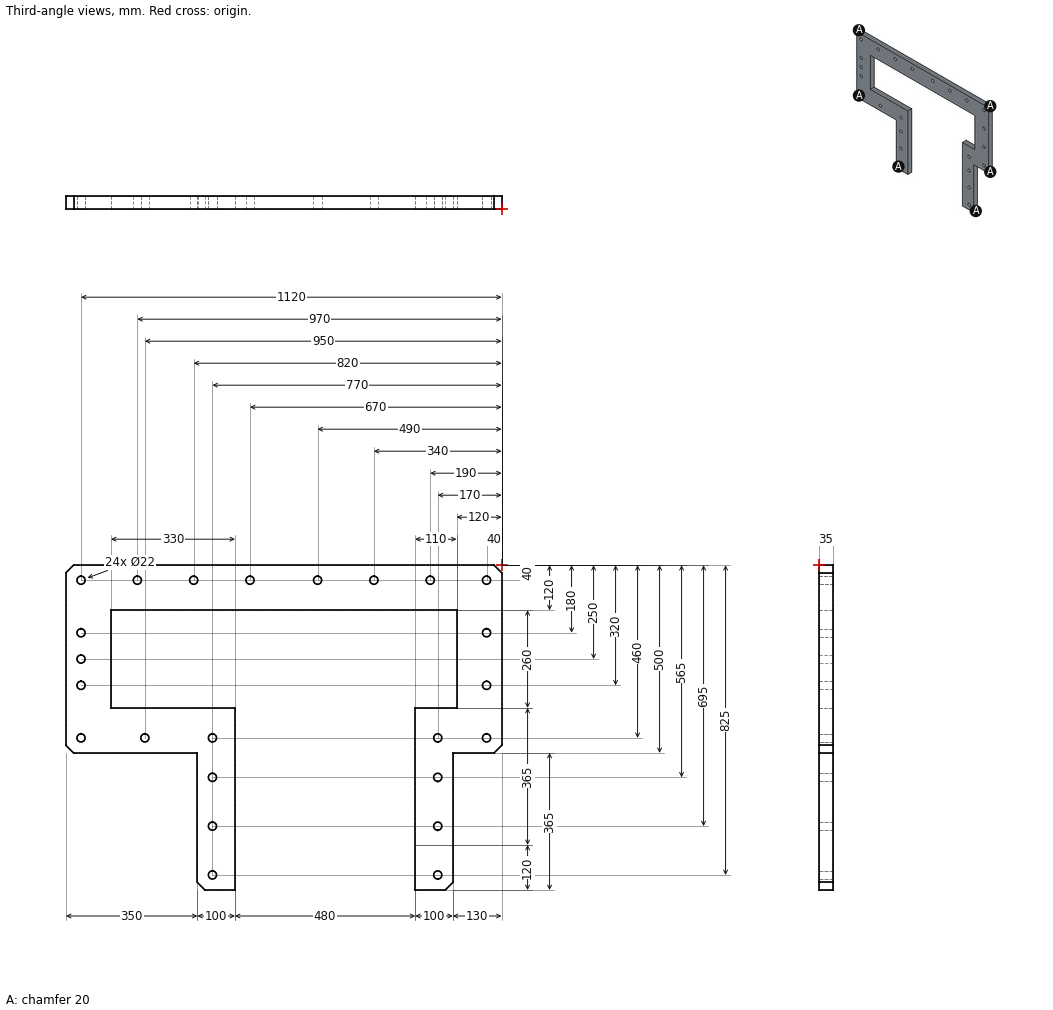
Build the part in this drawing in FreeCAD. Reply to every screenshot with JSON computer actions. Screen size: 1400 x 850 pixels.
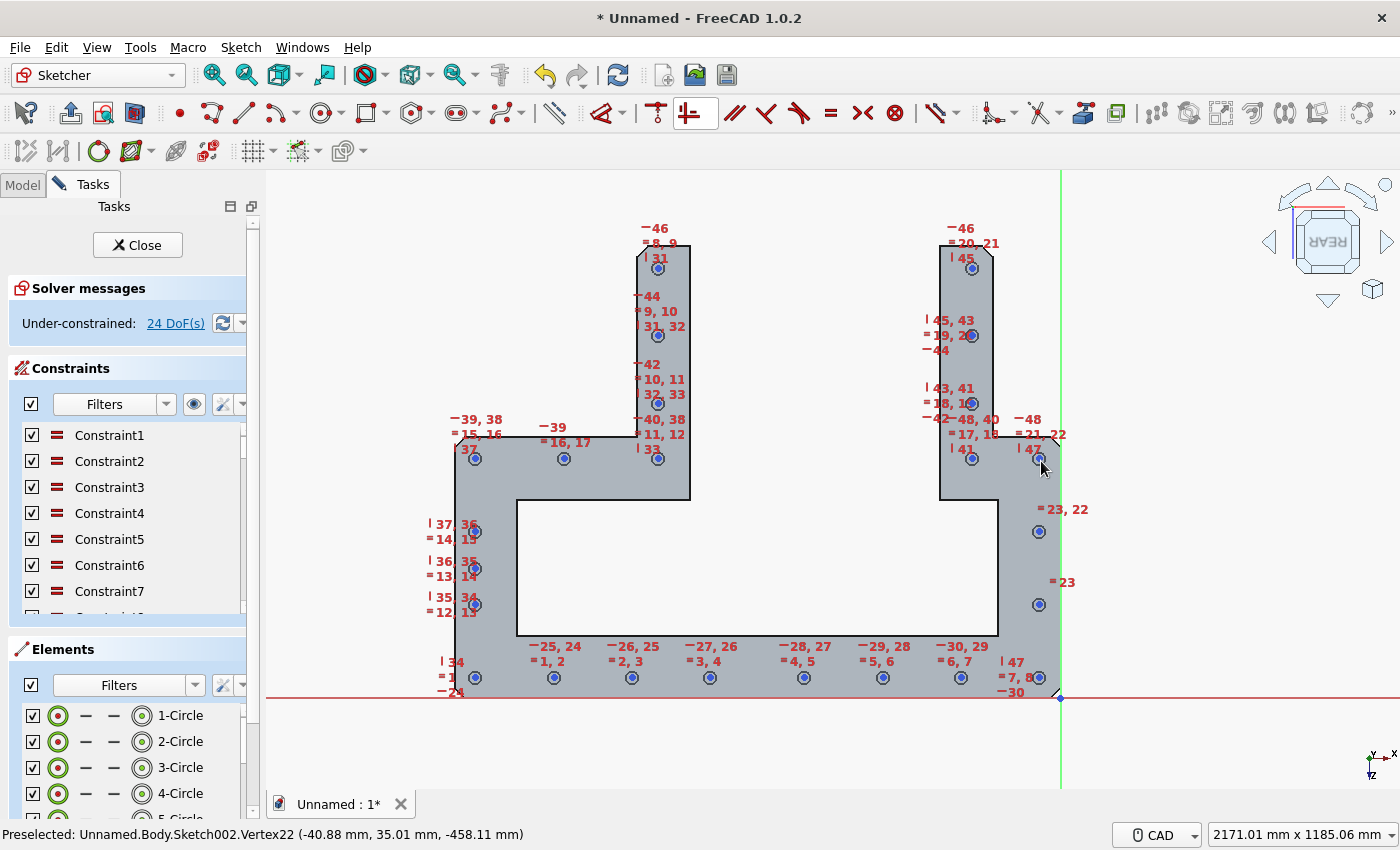
{"action": "left_click", "coordinate": [1039, 459]}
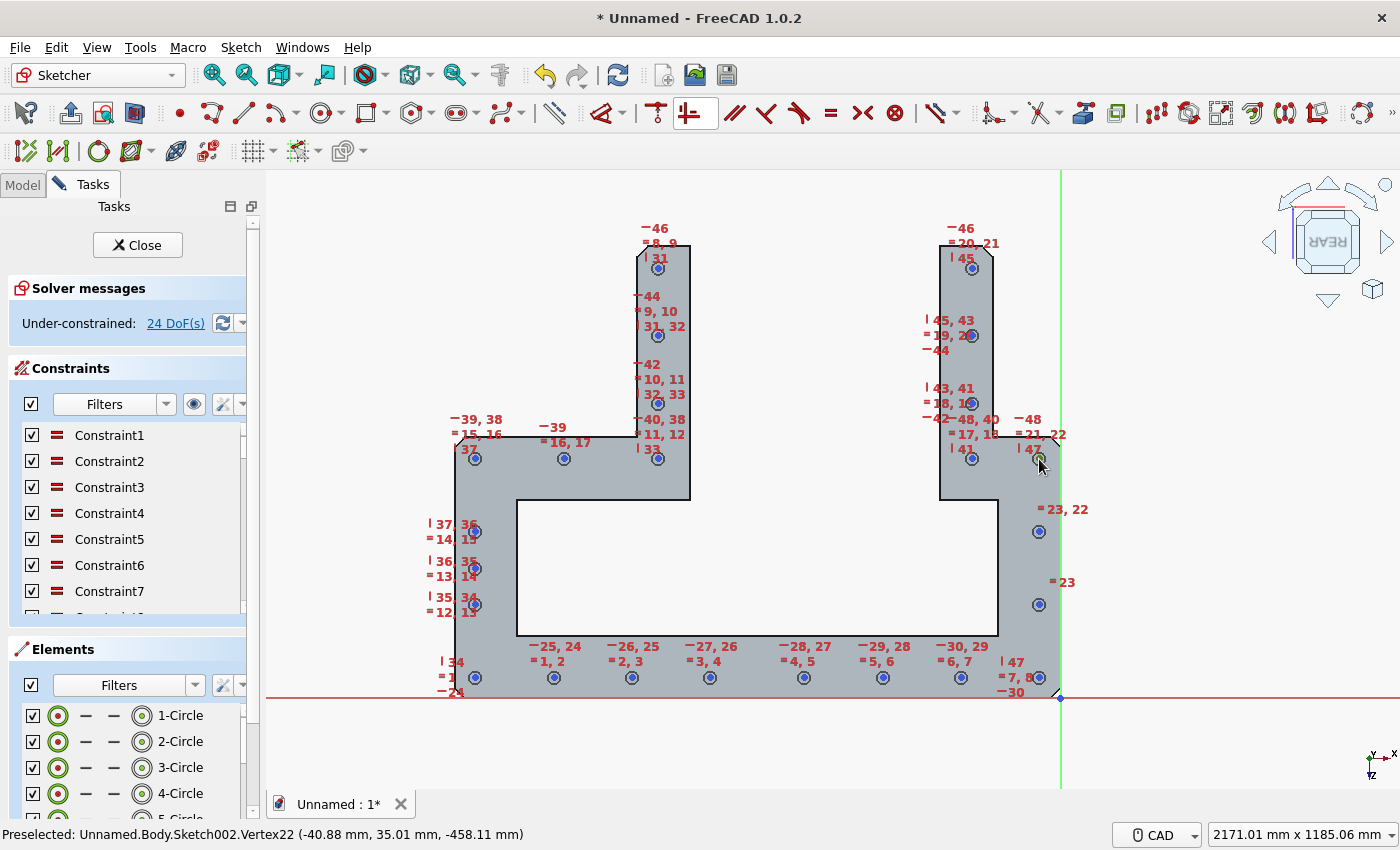
{"action": "left_click", "coordinate": [1039, 532]}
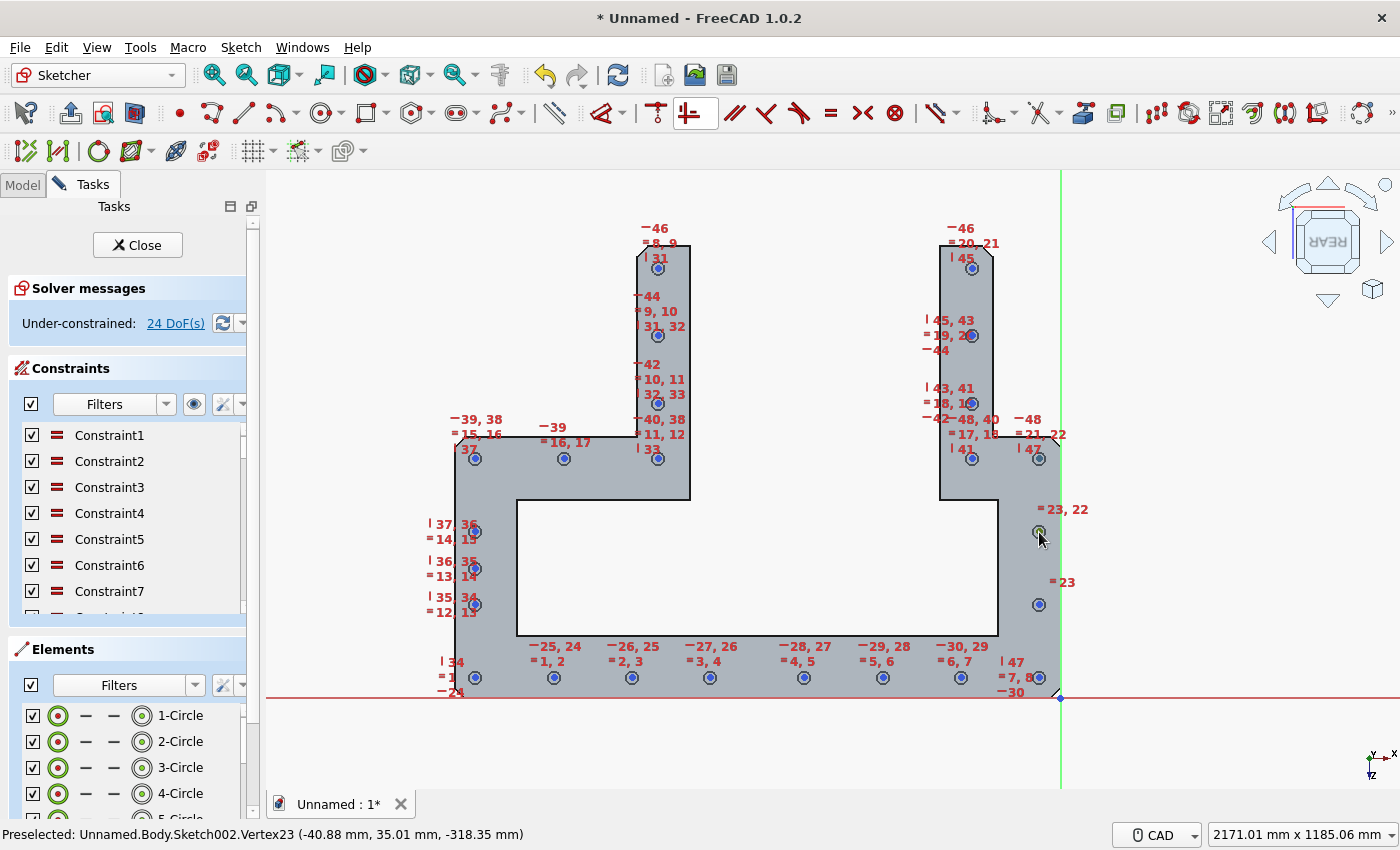
{"action": "key", "text": "v"}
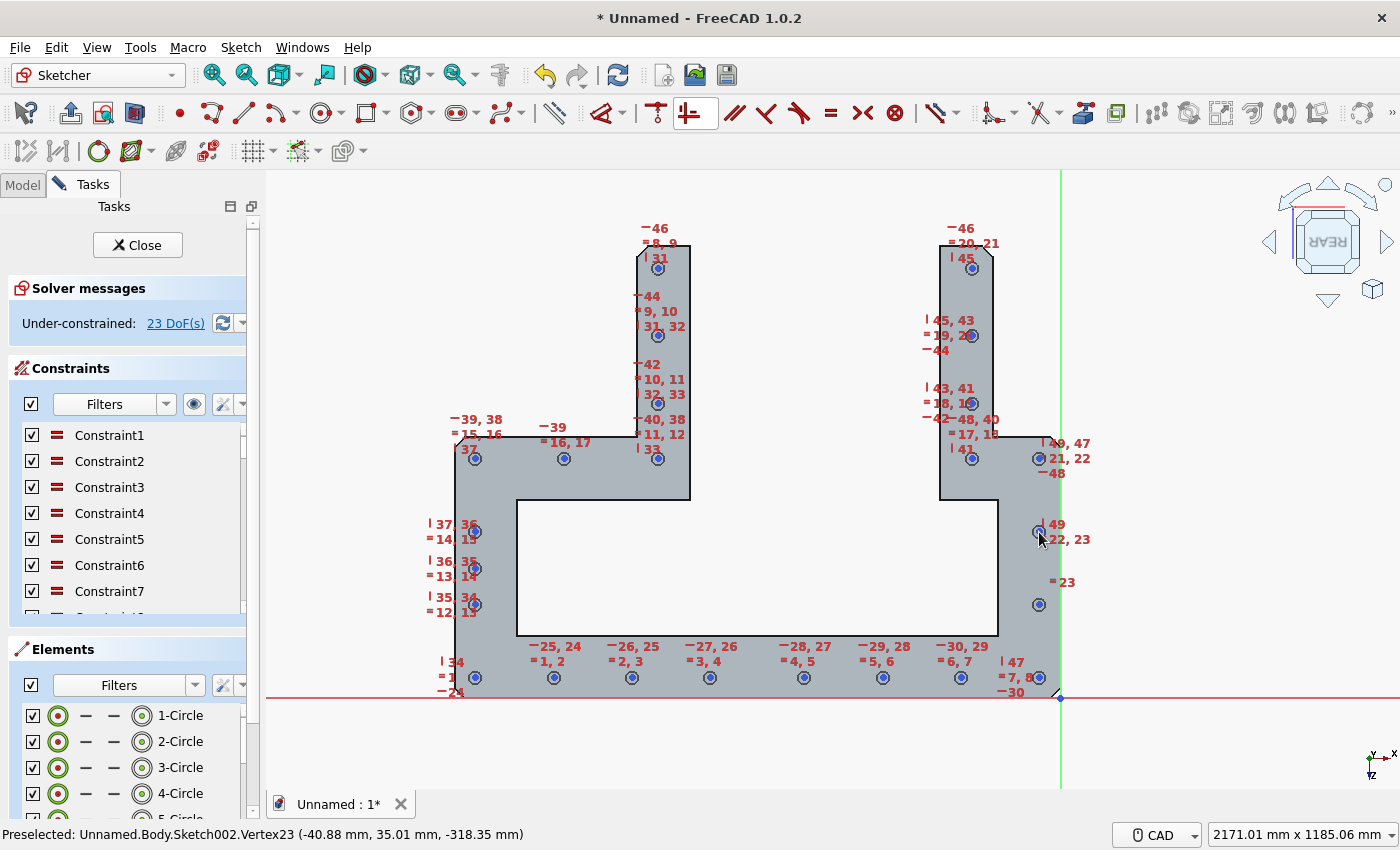
{"action": "left_click", "coordinate": [1039, 678]}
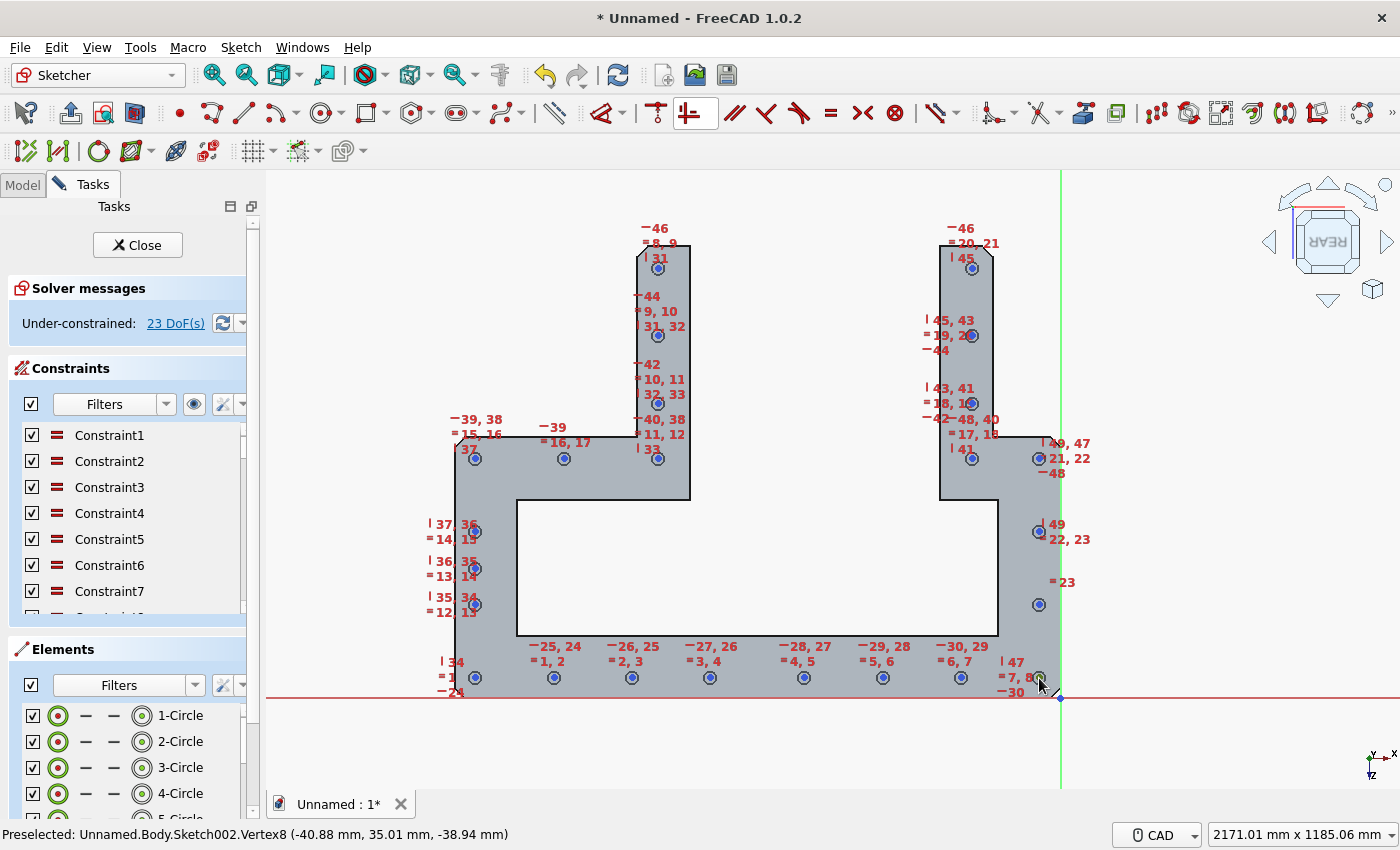
{"action": "left_click", "coordinate": [1039, 605]}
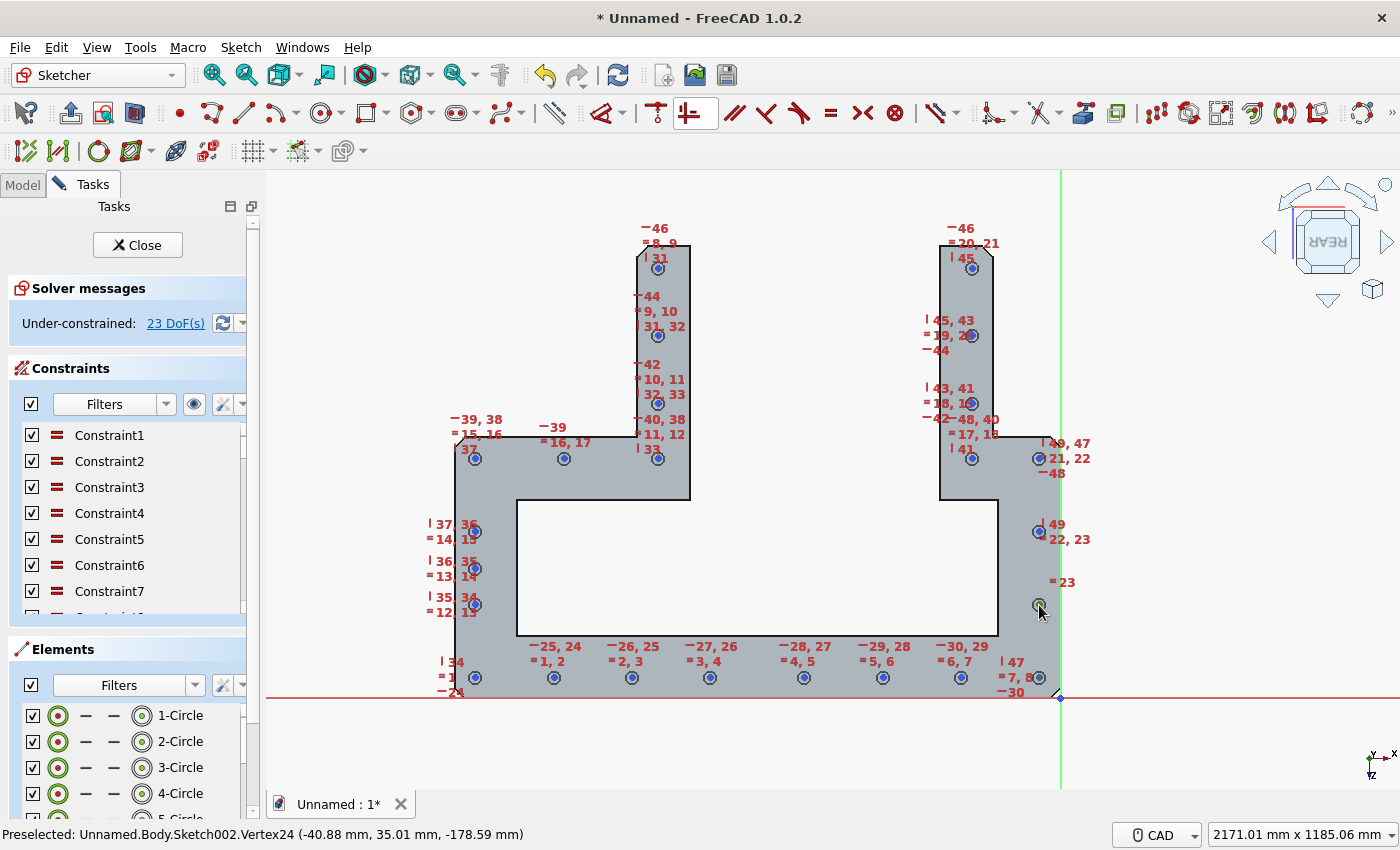
{"action": "key", "text": "v"}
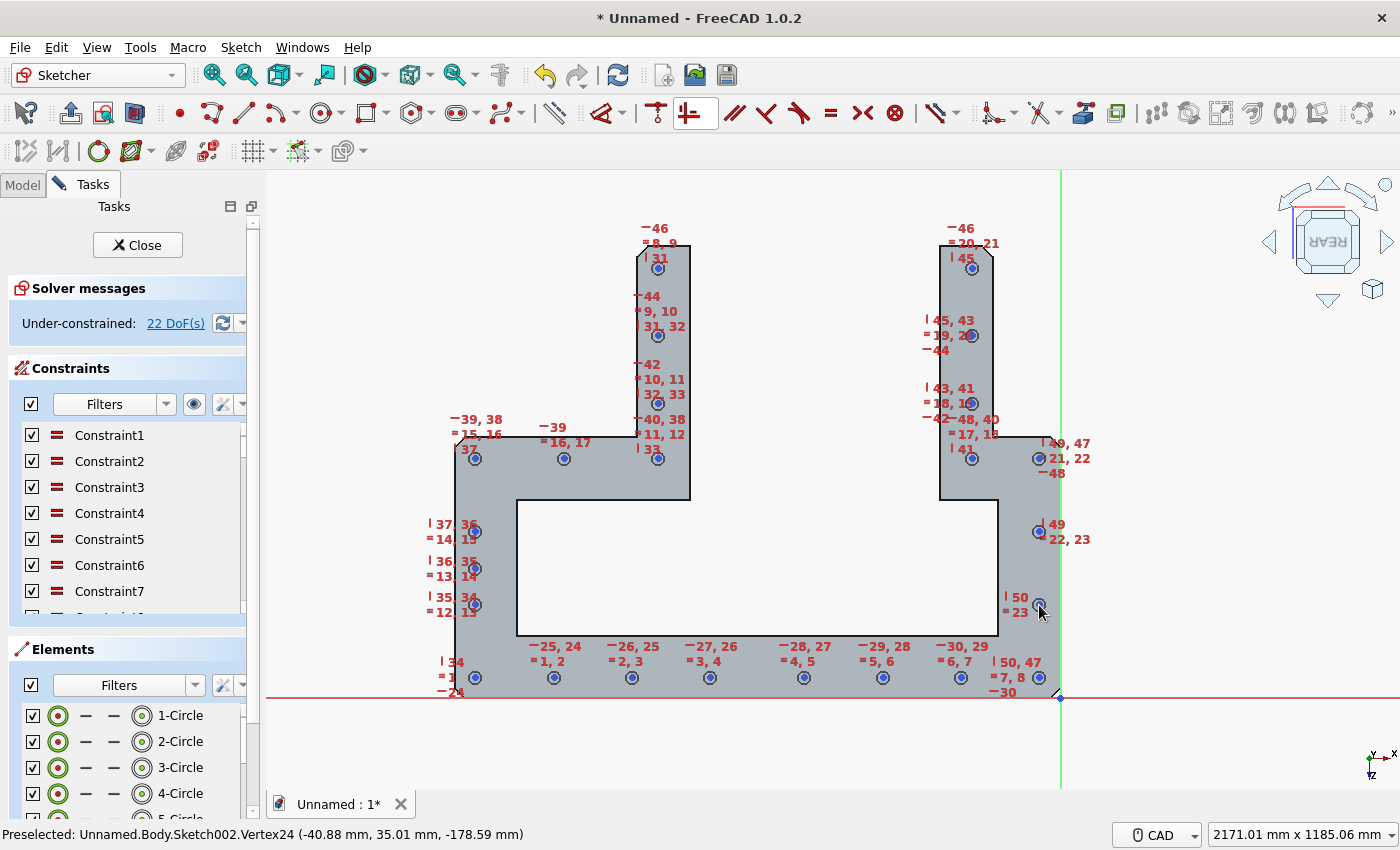
{"action": "left_click", "coordinate": [602, 114]}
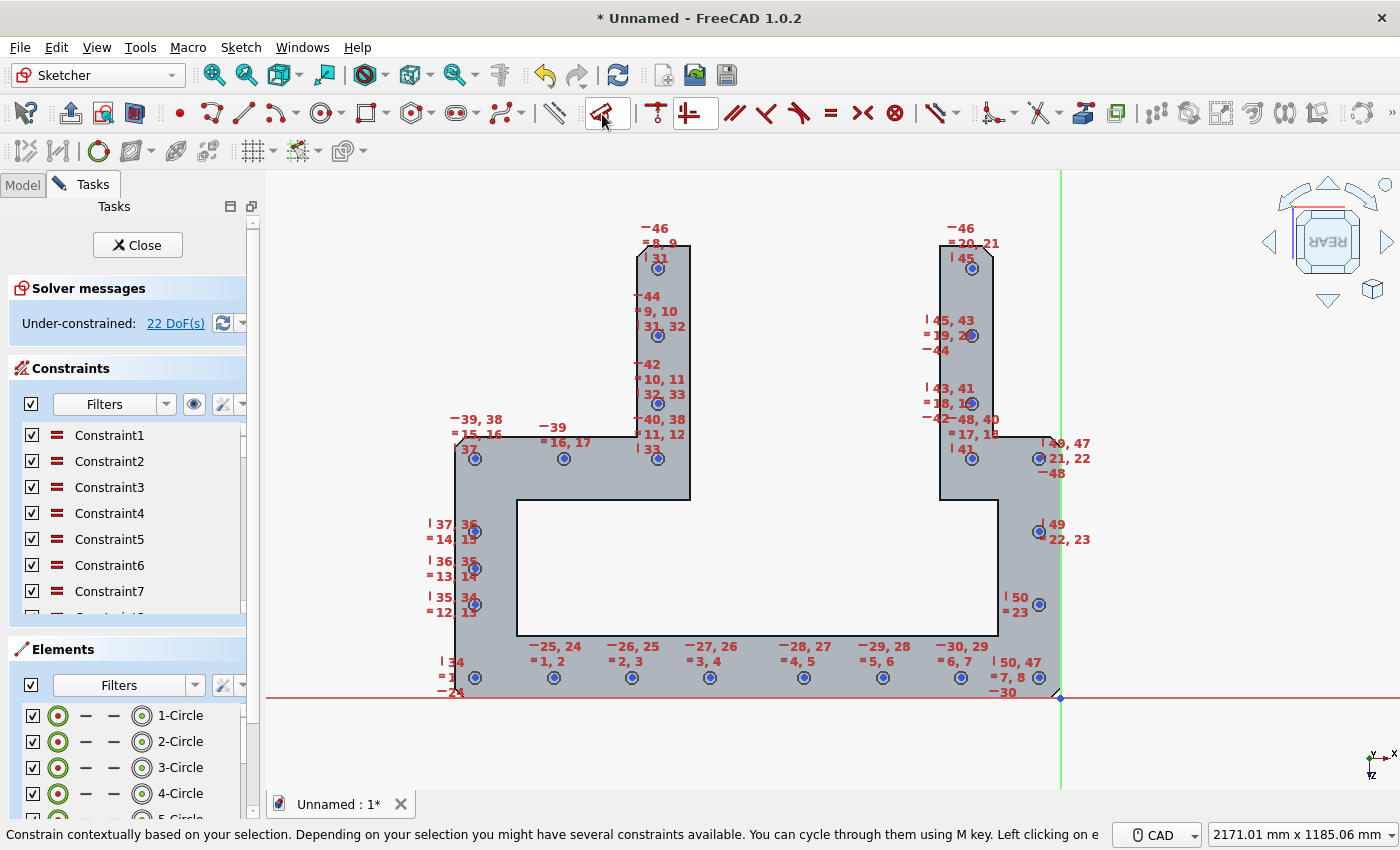
{"action": "scroll", "coordinate": [469, 678], "scroll_direction": "up", "scroll_amount": 7}